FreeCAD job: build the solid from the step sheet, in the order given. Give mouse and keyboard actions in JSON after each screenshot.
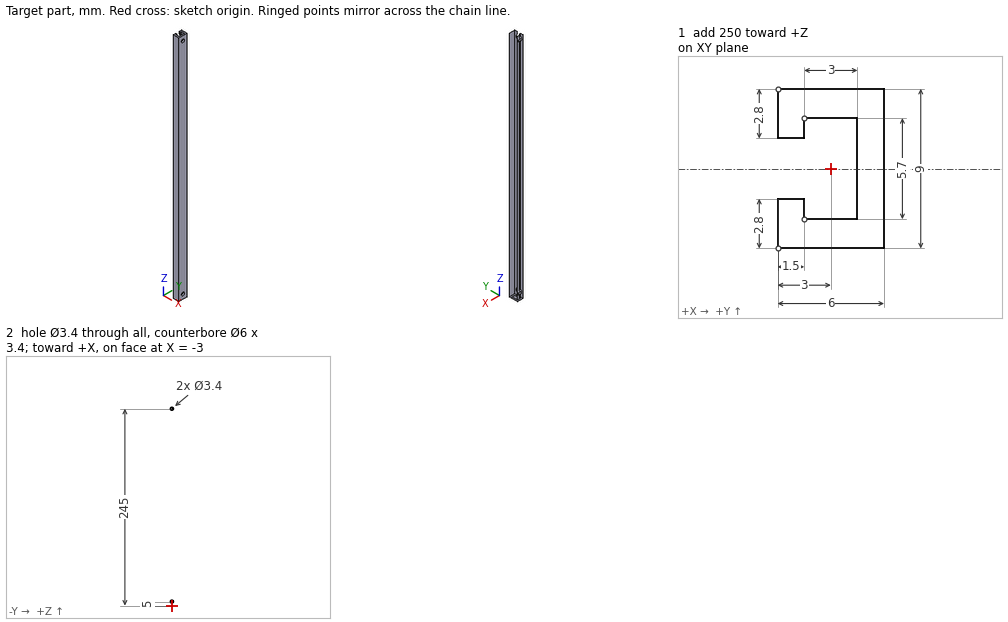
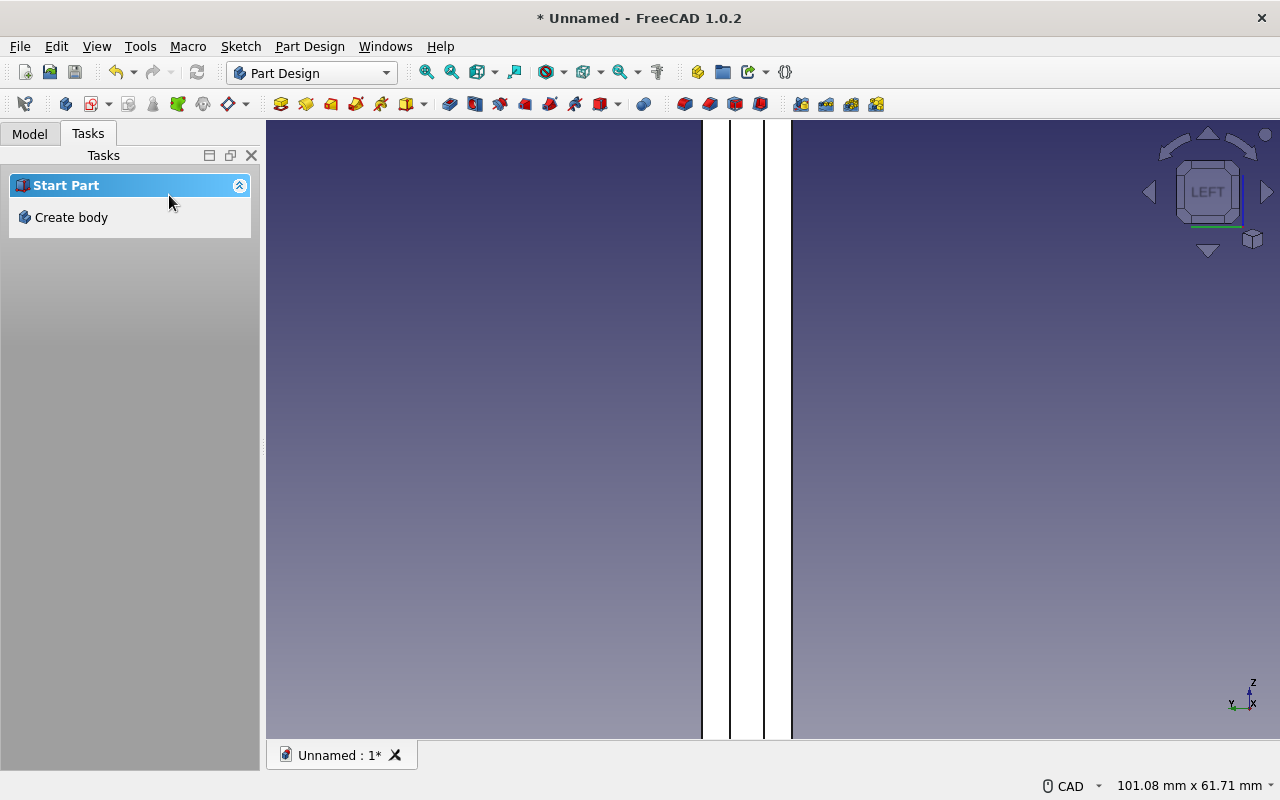
{"action": "key", "text": "0"}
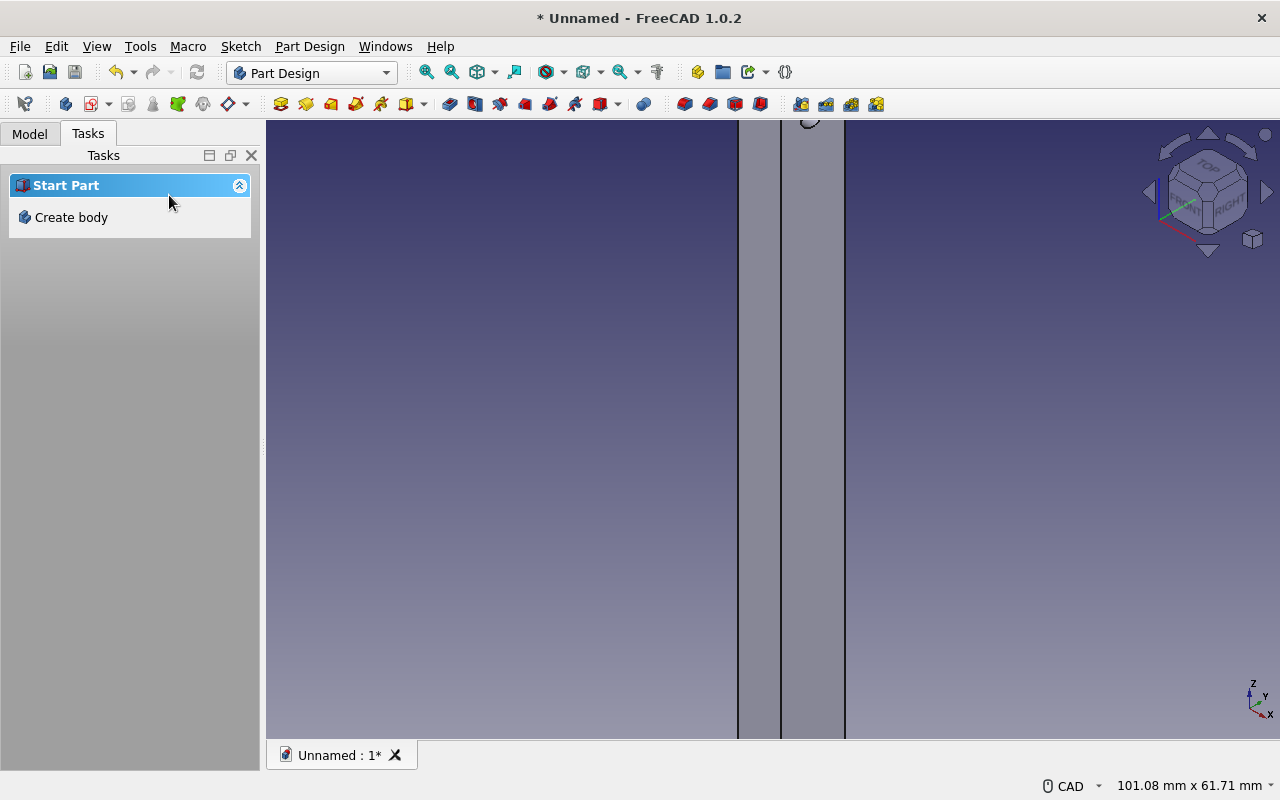
{"action": "left_click", "coordinate": [427, 72]}